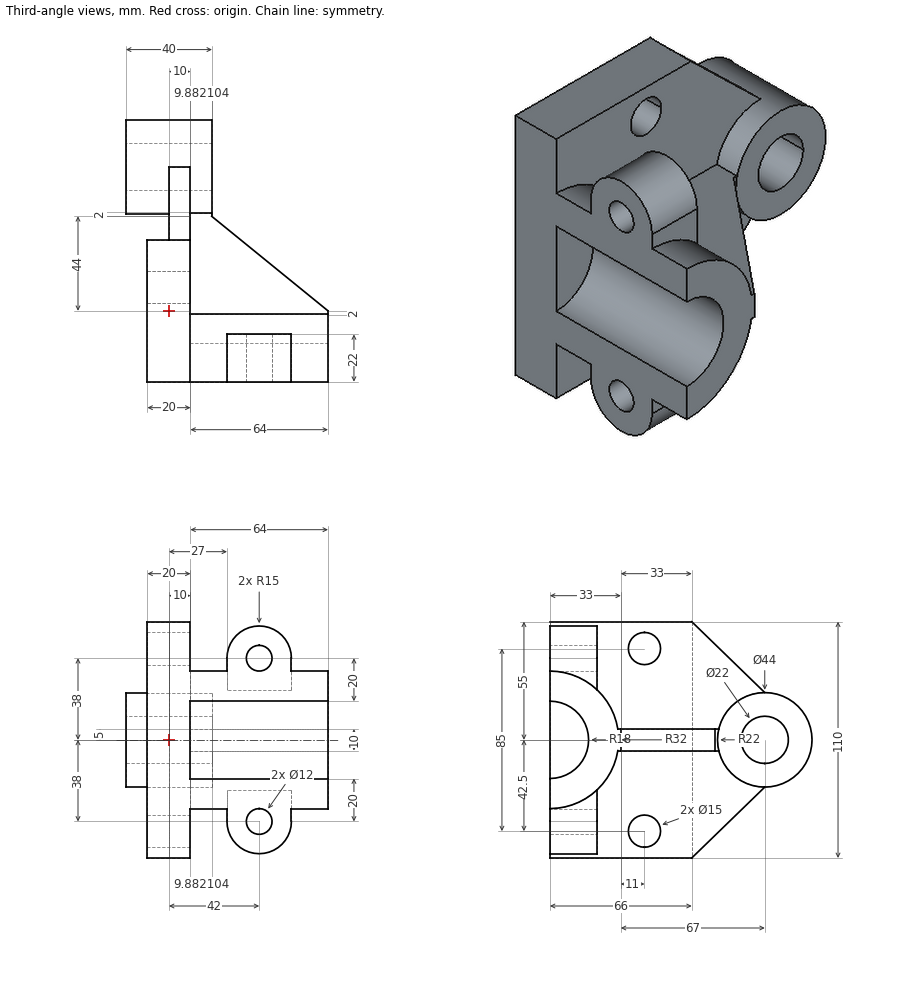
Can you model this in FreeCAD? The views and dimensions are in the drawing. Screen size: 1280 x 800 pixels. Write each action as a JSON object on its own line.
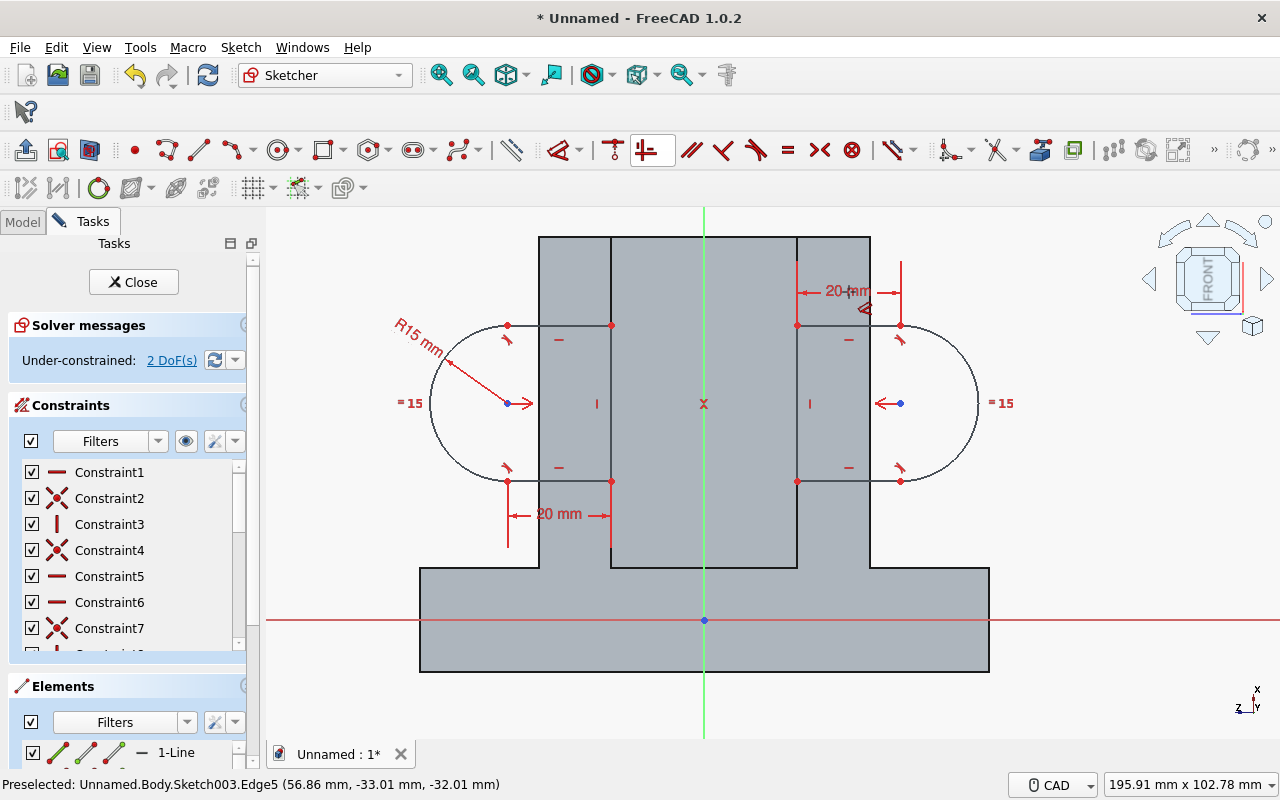
{"action": "left_click", "coordinate": [508, 481]}
{"action": "left_click", "coordinate": [606, 654]}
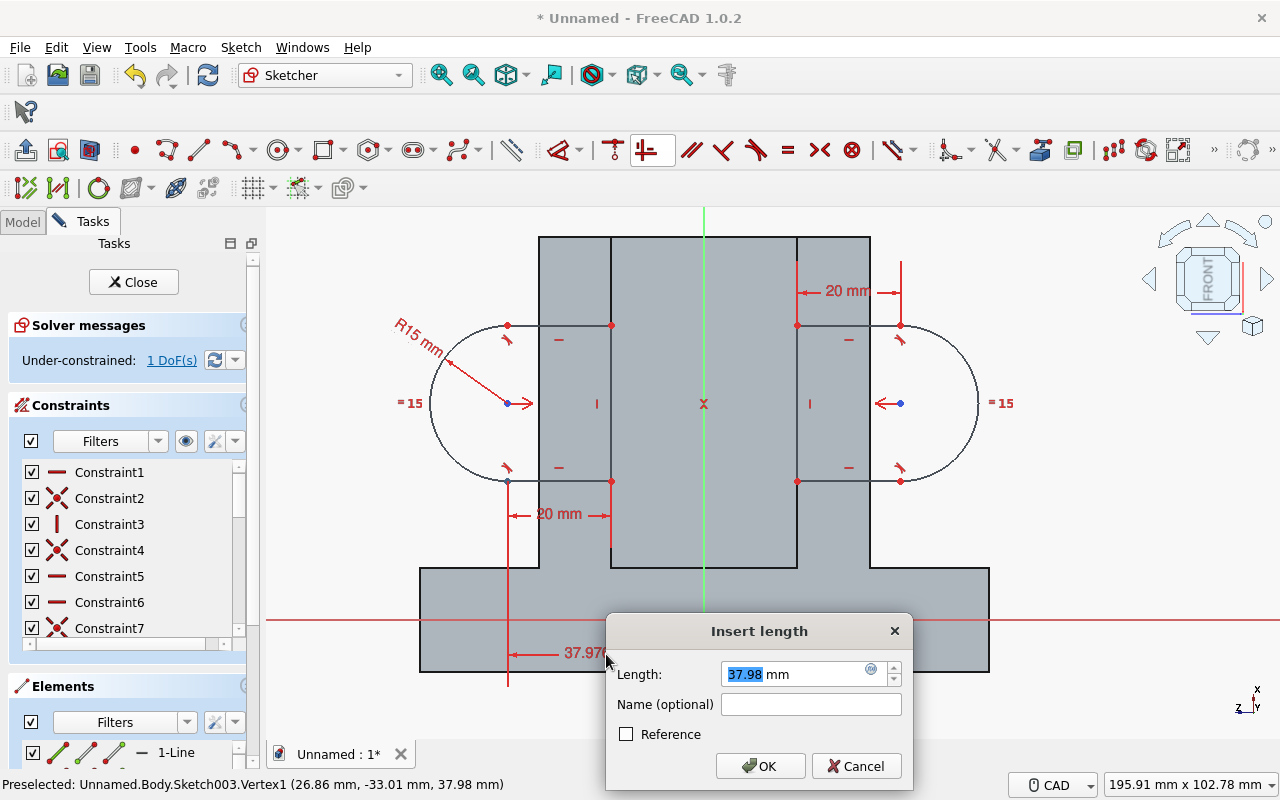
{"action": "type", "text": "38"}
{"action": "key", "text": "Return"}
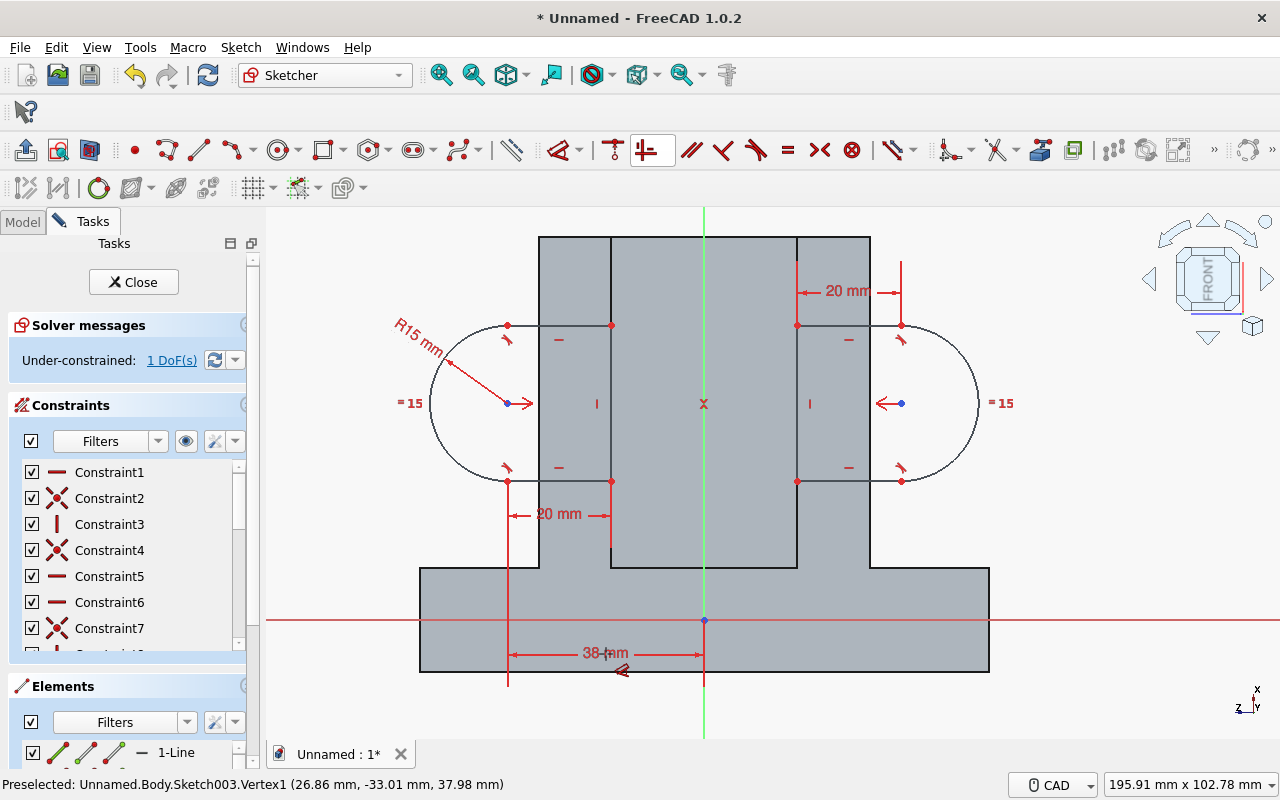
{"action": "left_click", "coordinate": [508, 481]}
{"action": "left_click", "coordinate": [474, 551]}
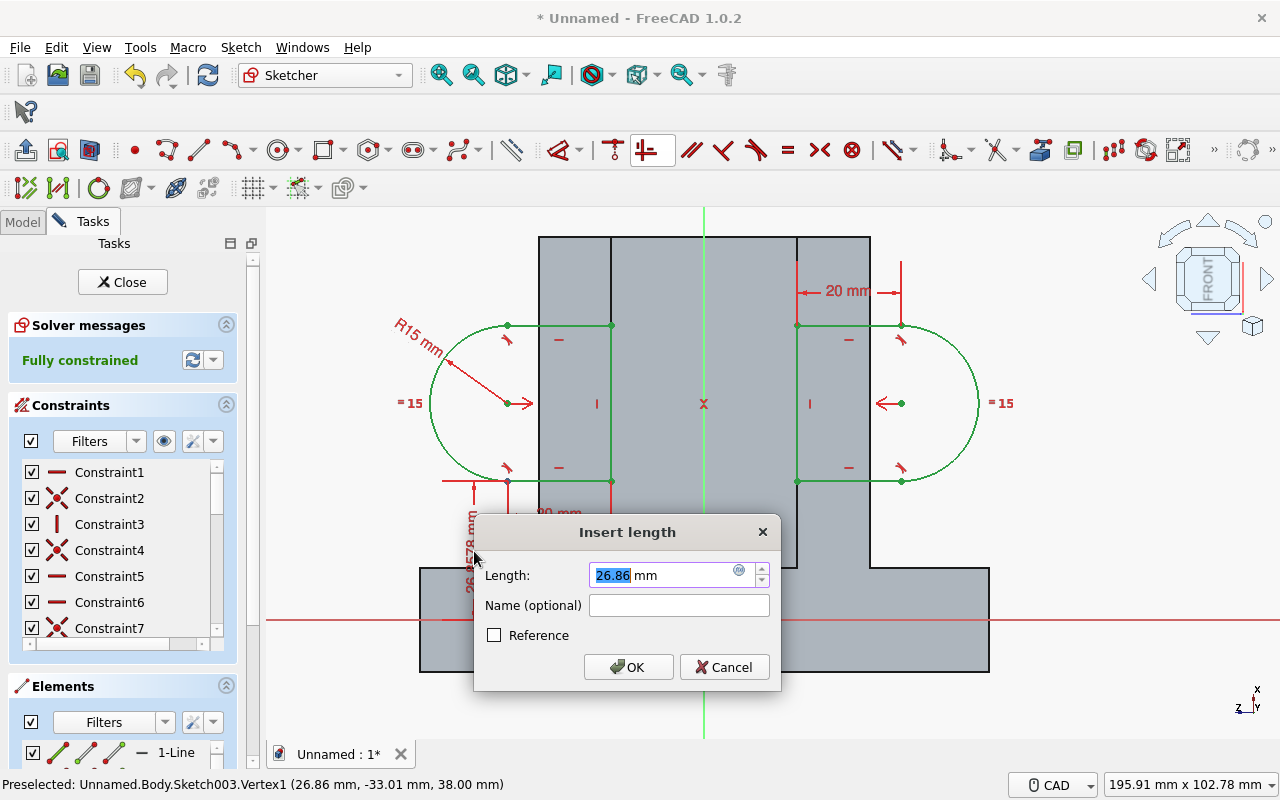
{"action": "type", "text": "27"}
{"action": "key", "text": "Return"}
{"action": "key", "text": "Escape"}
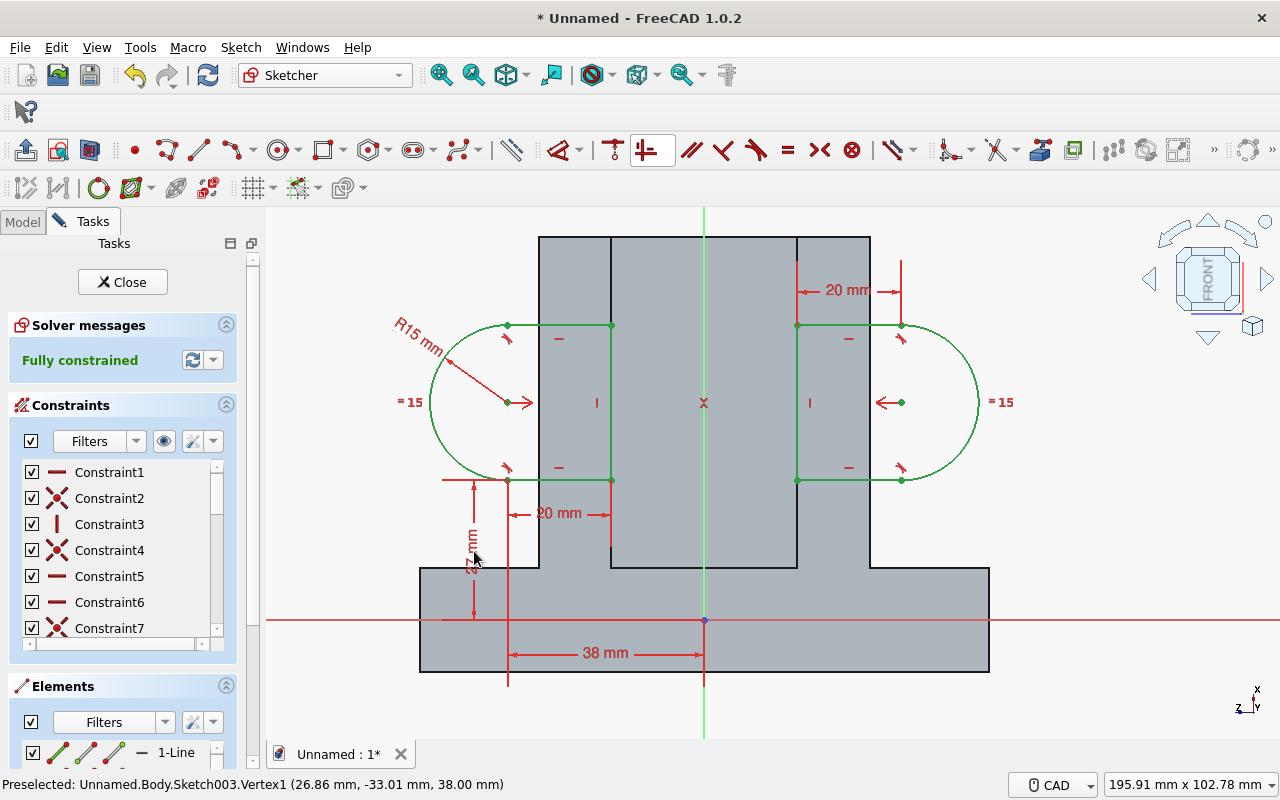
{"action": "left_click", "coordinate": [123, 282]}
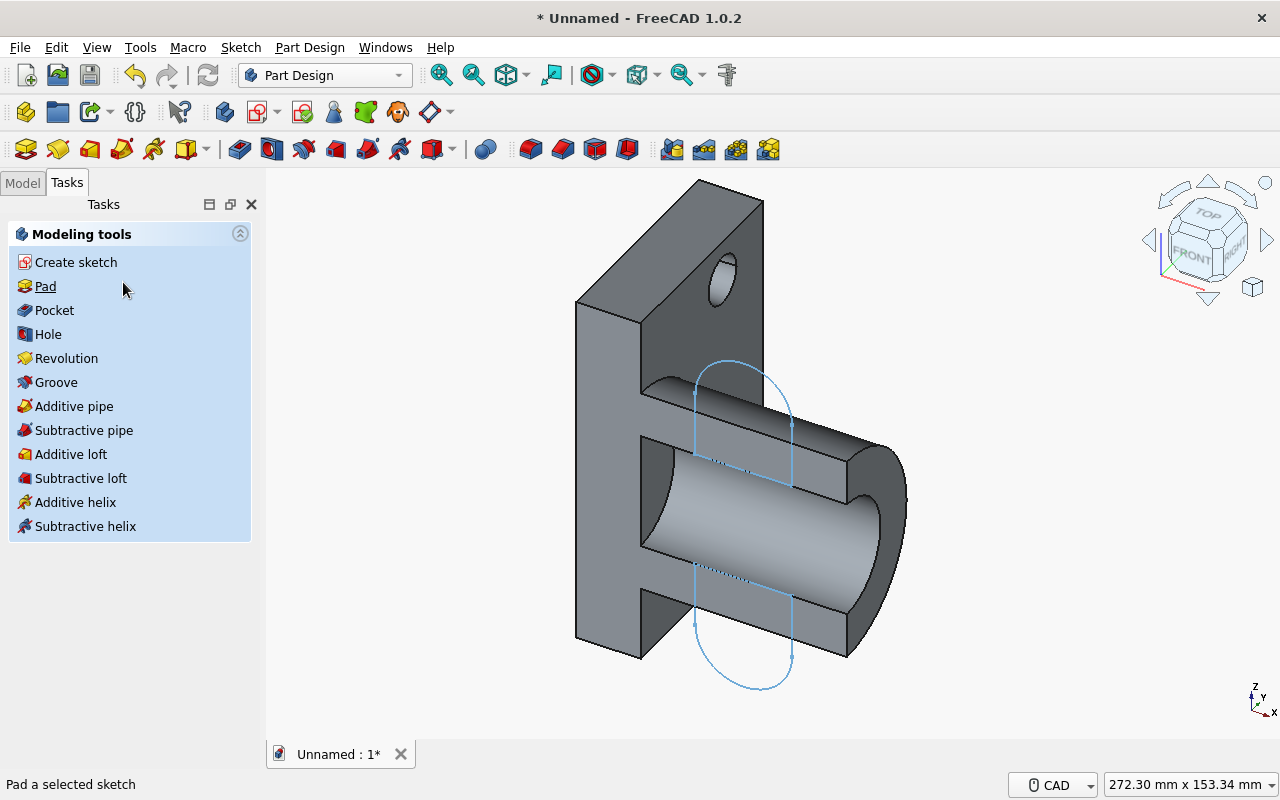
{"action": "left_click", "coordinate": [26, 150]}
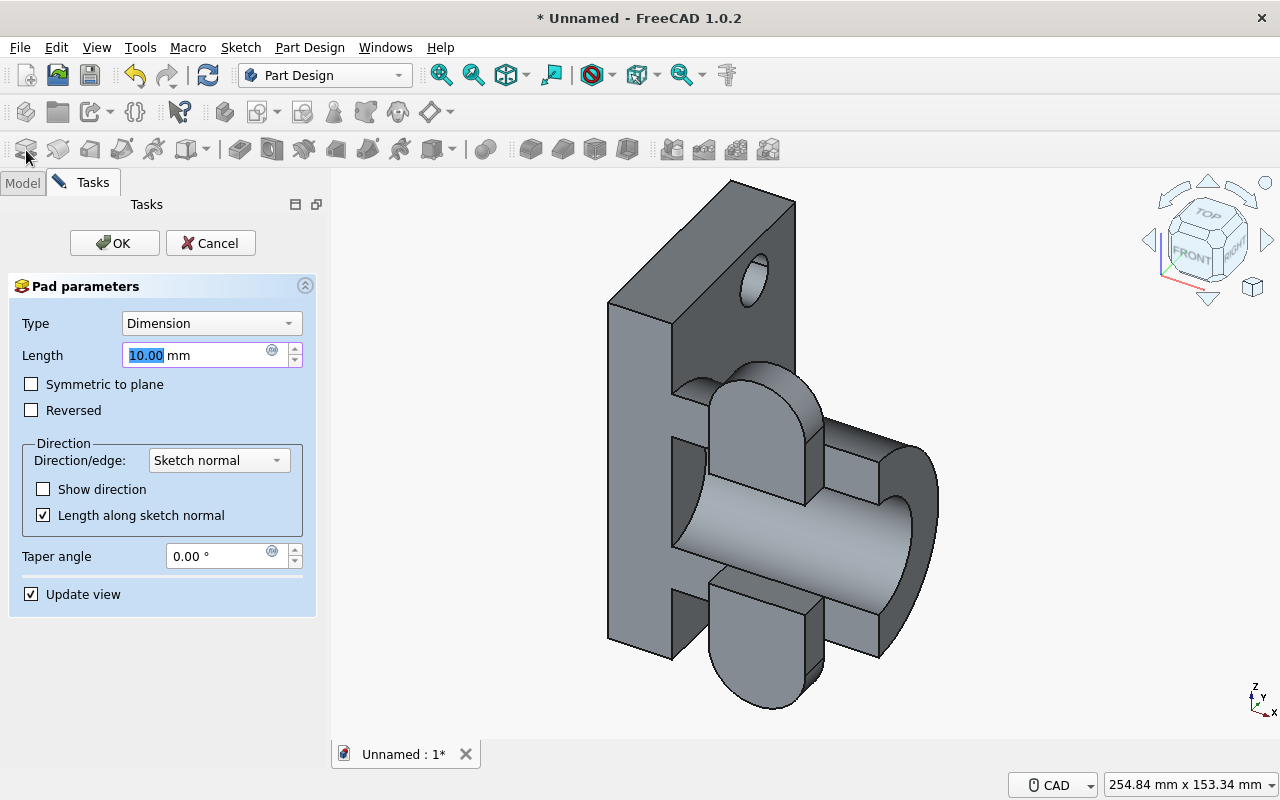
{"action": "type", "text": "22"}
{"action": "key", "text": "Tab"}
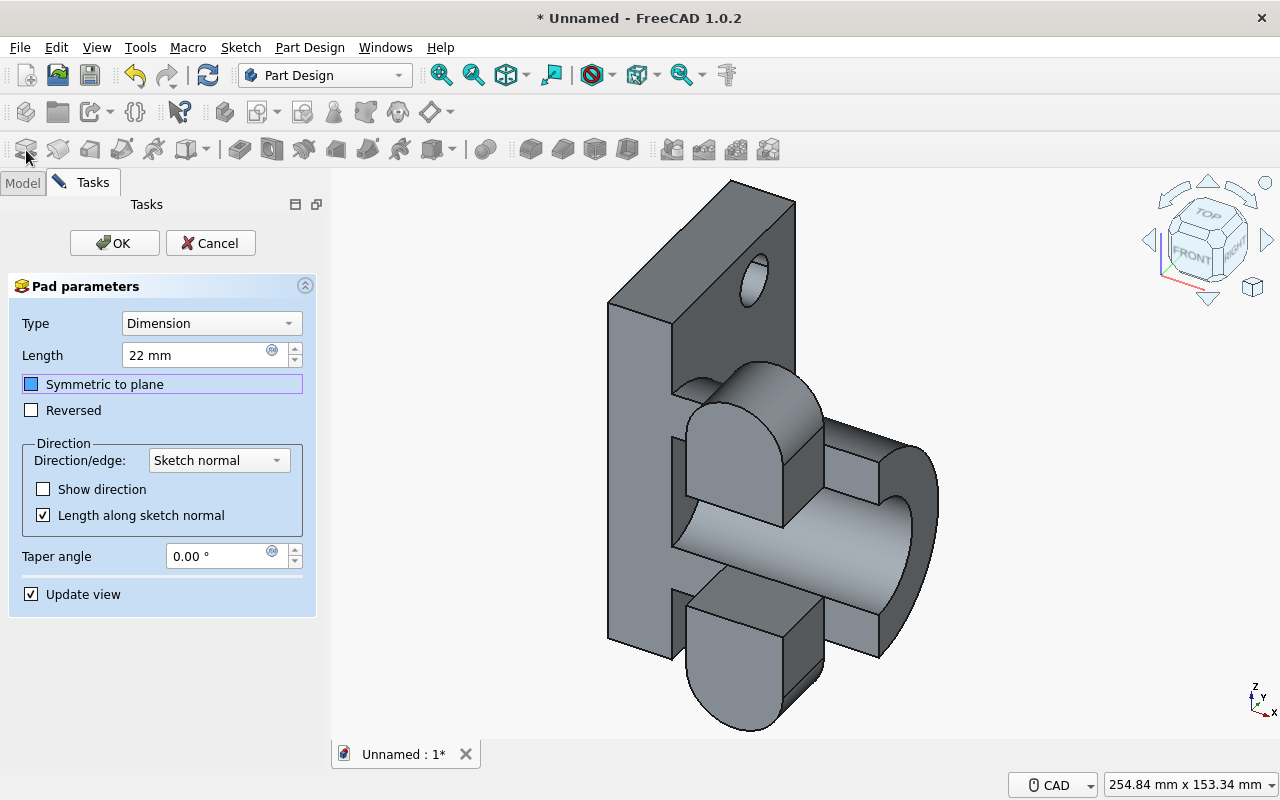
{"action": "left_click", "coordinate": [30, 410]}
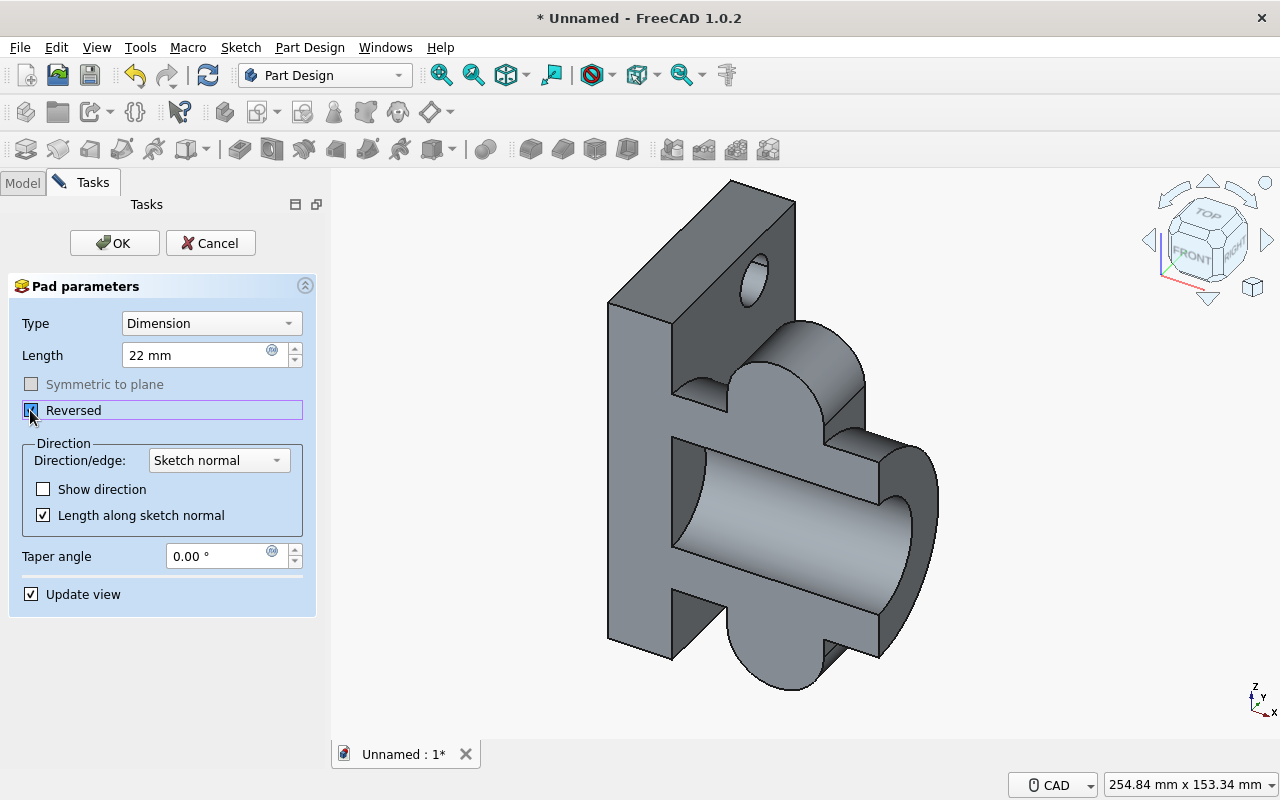
{"action": "left_click", "coordinate": [115, 243]}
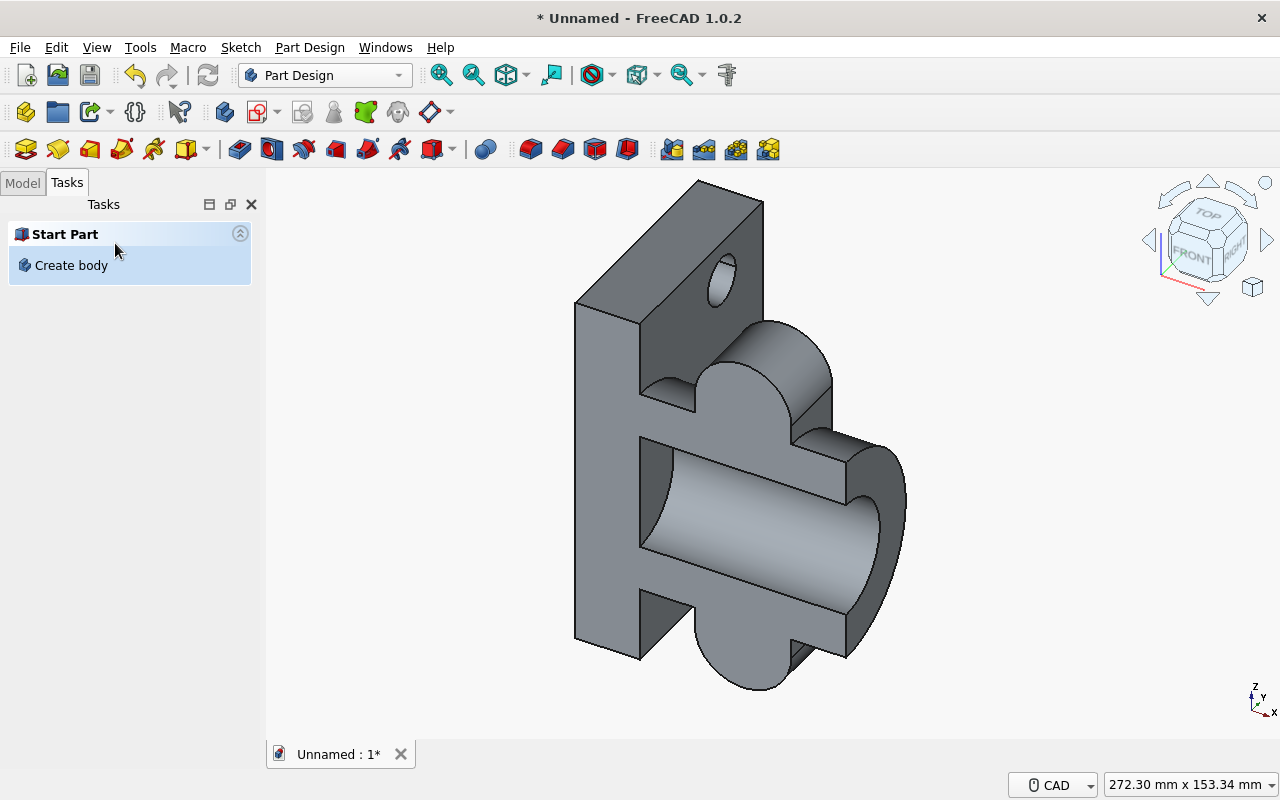
{"action": "key", "text": "4"}